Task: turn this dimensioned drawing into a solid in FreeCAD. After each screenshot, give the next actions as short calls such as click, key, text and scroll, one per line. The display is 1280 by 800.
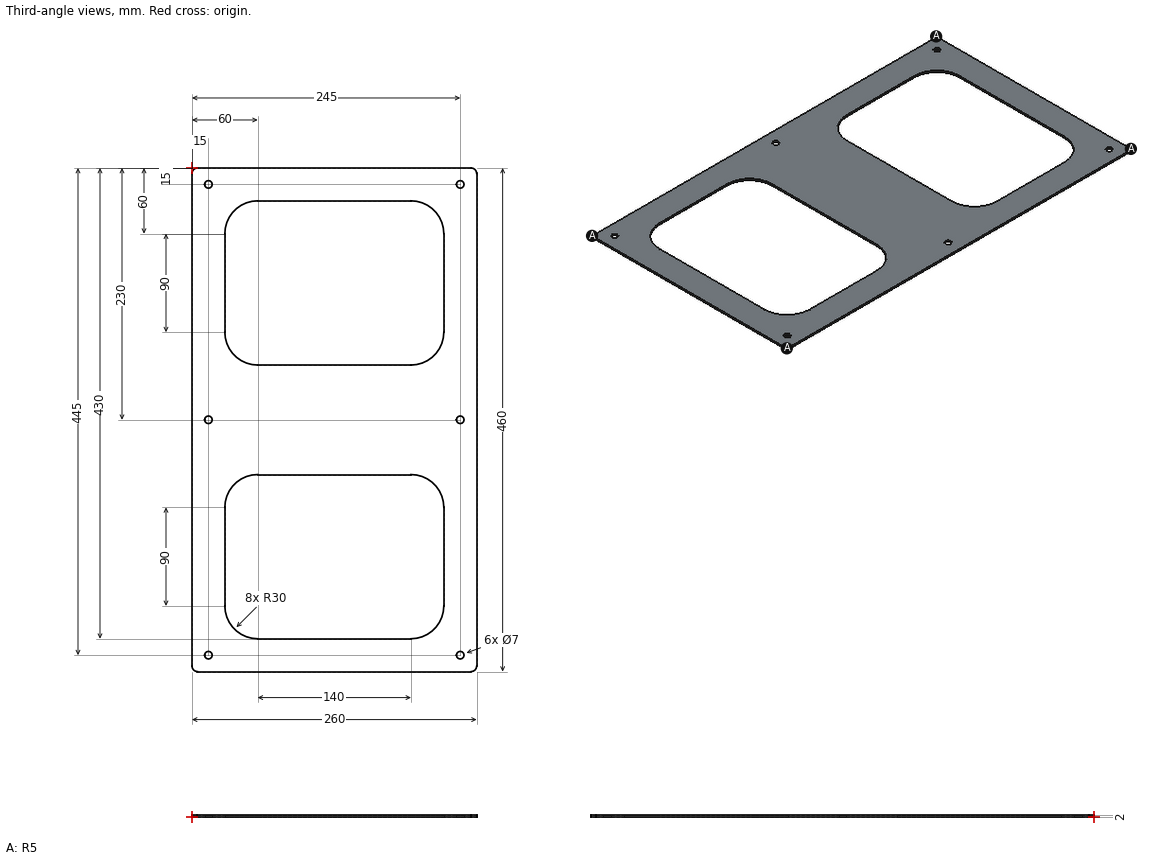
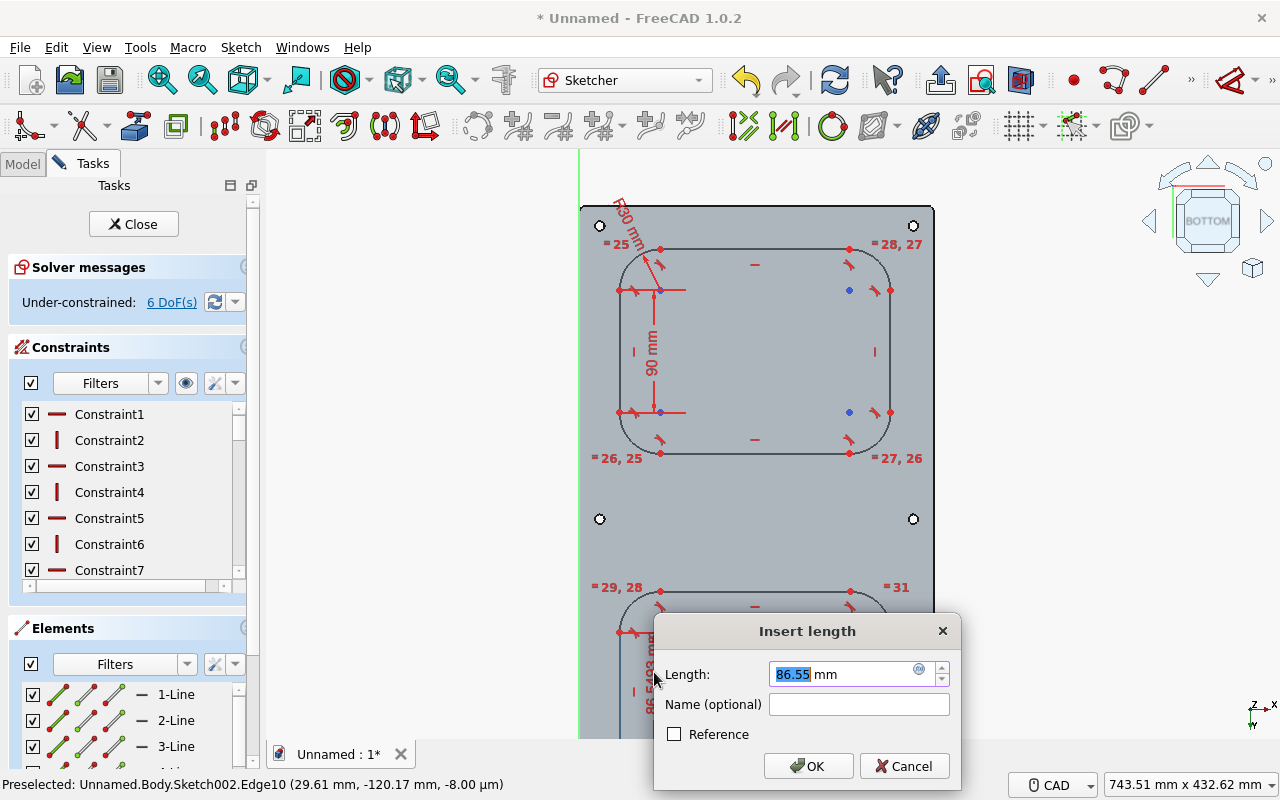
text(90)
key(Return)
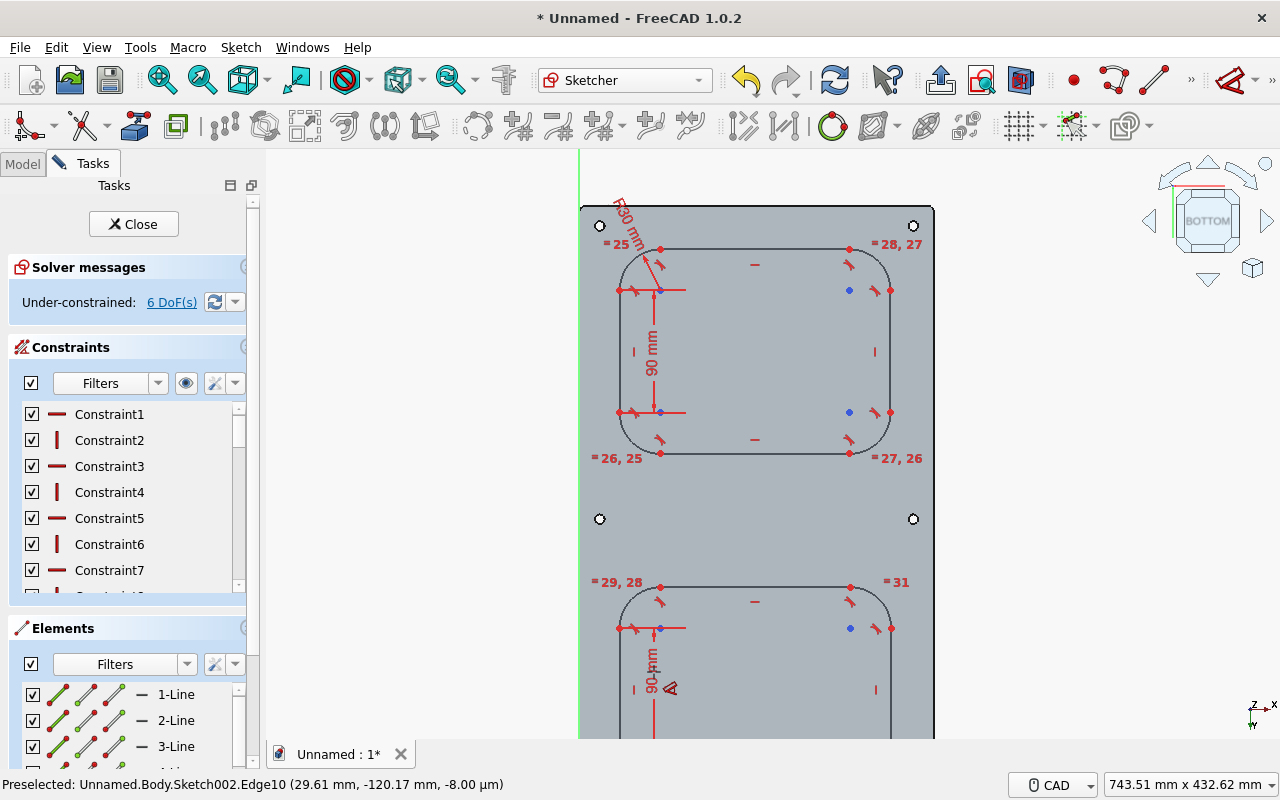
click(793, 249)
click(755, 215)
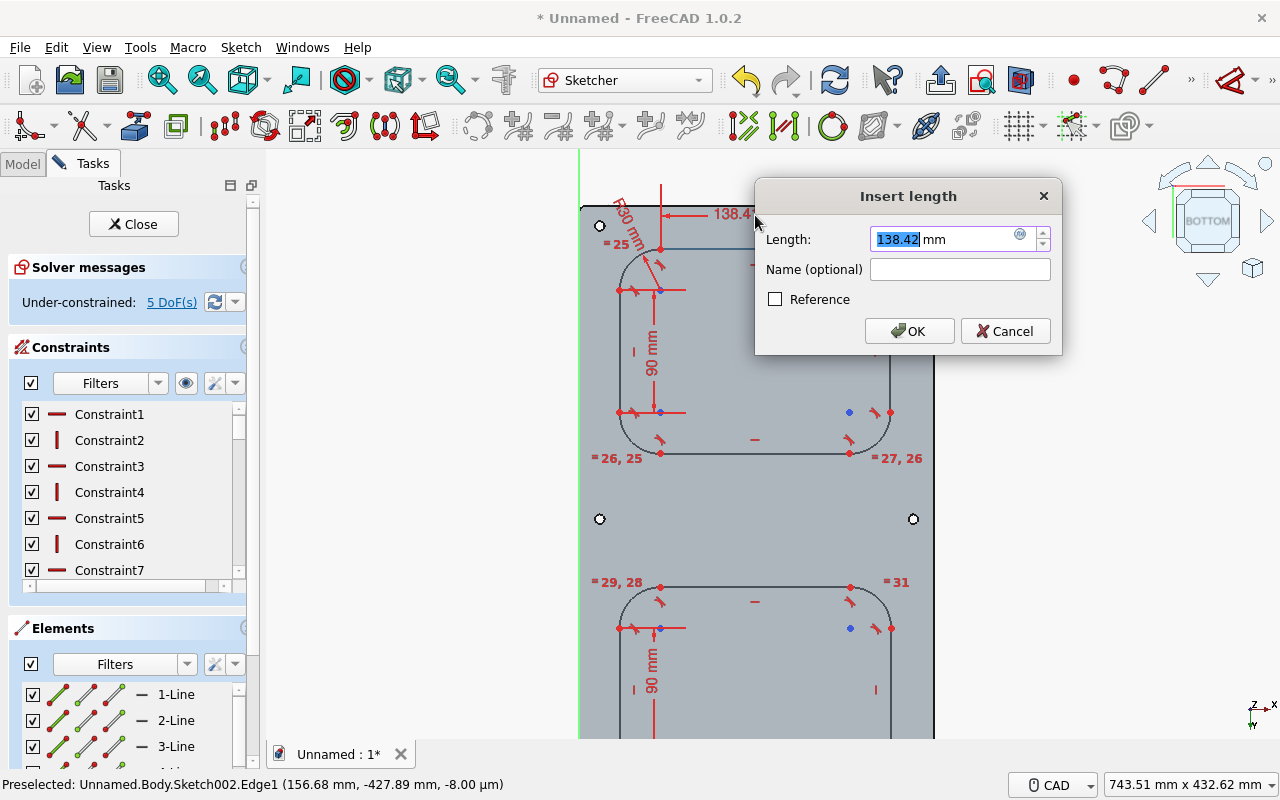
text(140)
key(Return)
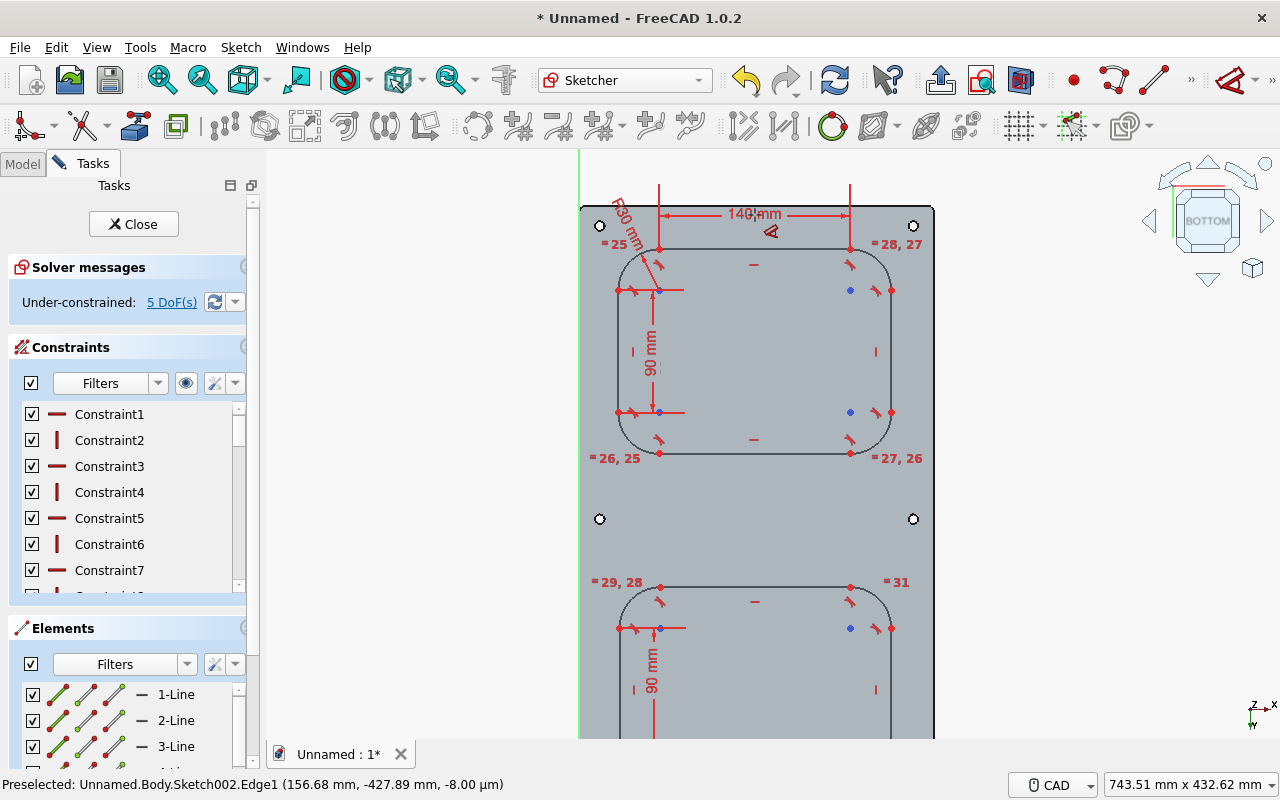
click(793, 587)
click(755, 621)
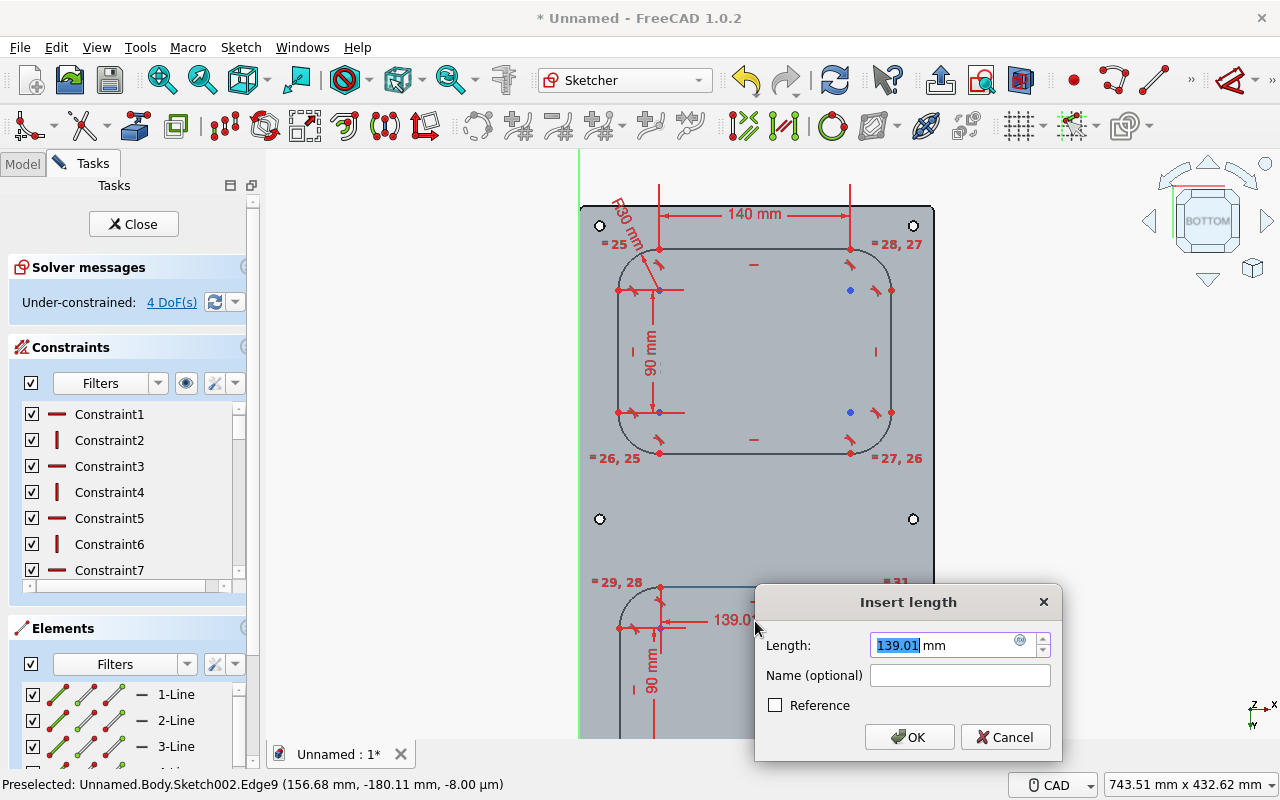
text(140)
key(Return)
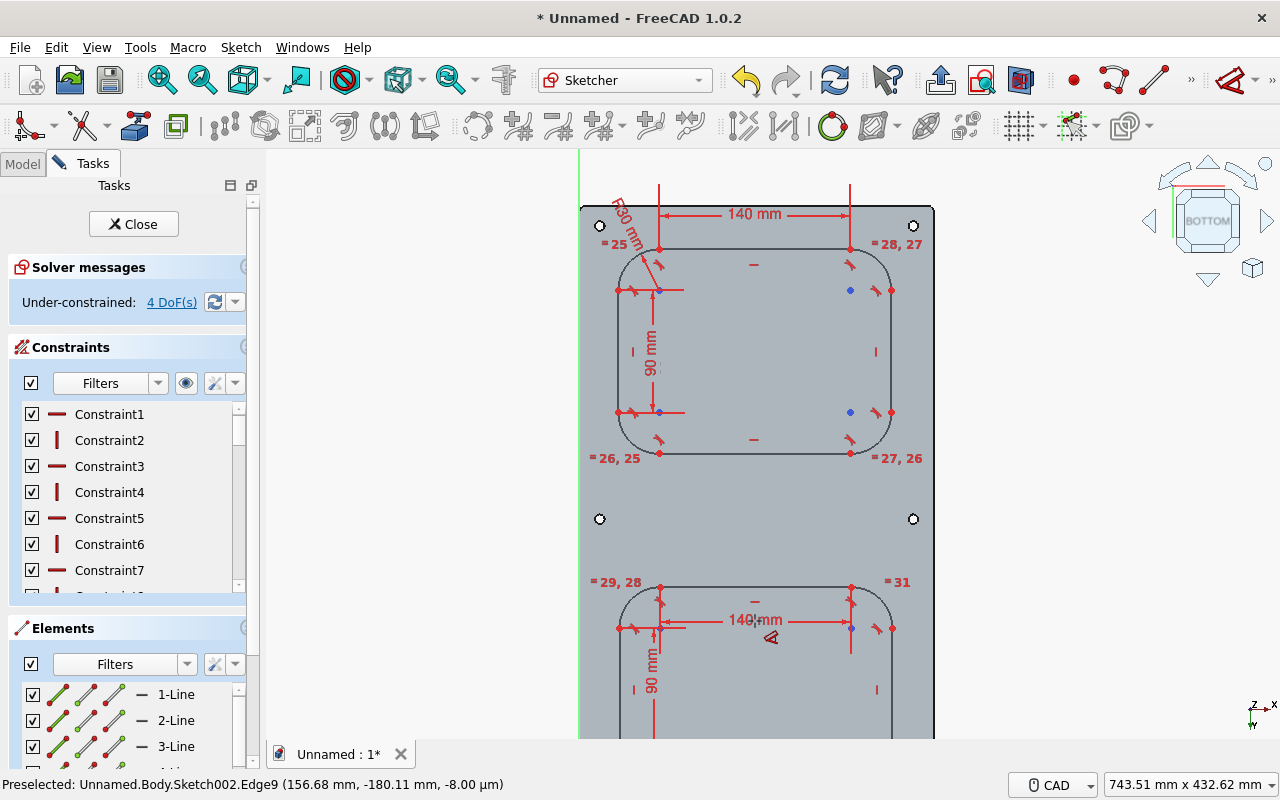
click(659, 249)
click(619, 191)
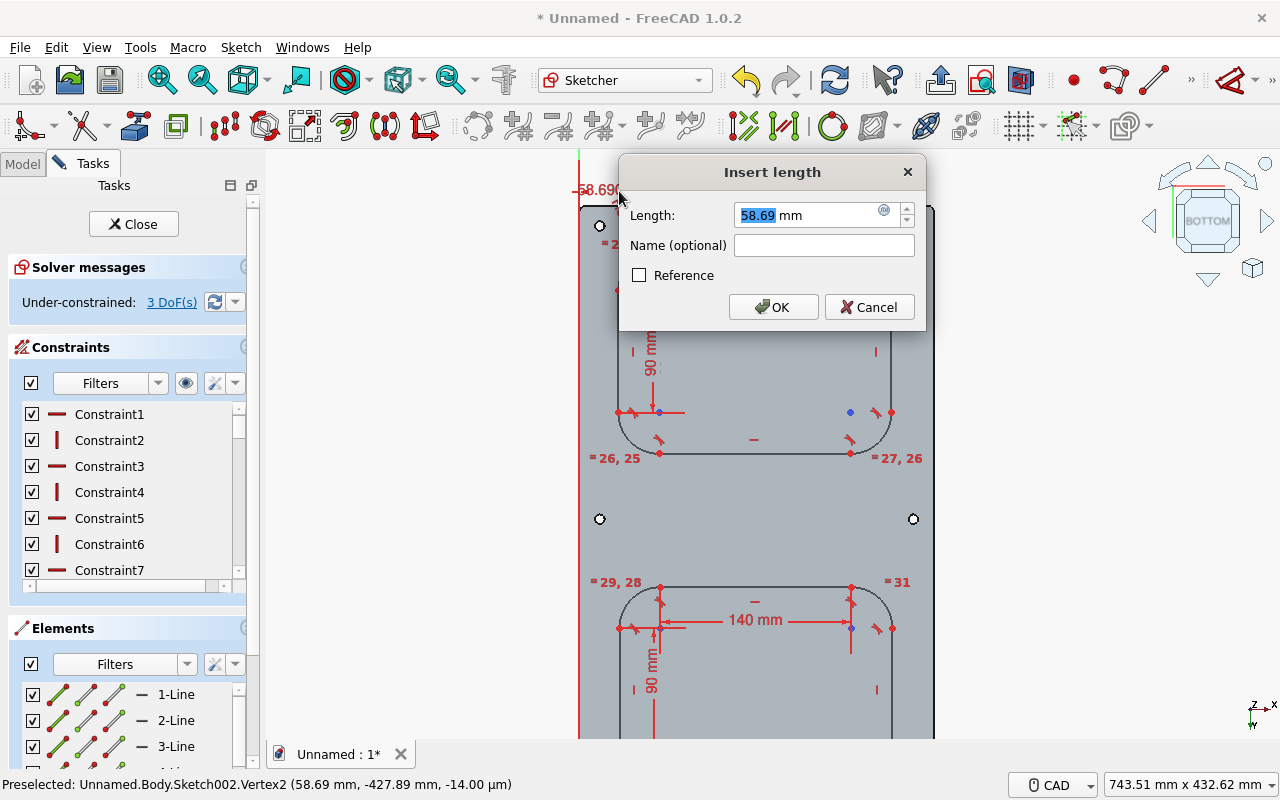
text(60)
key(Return)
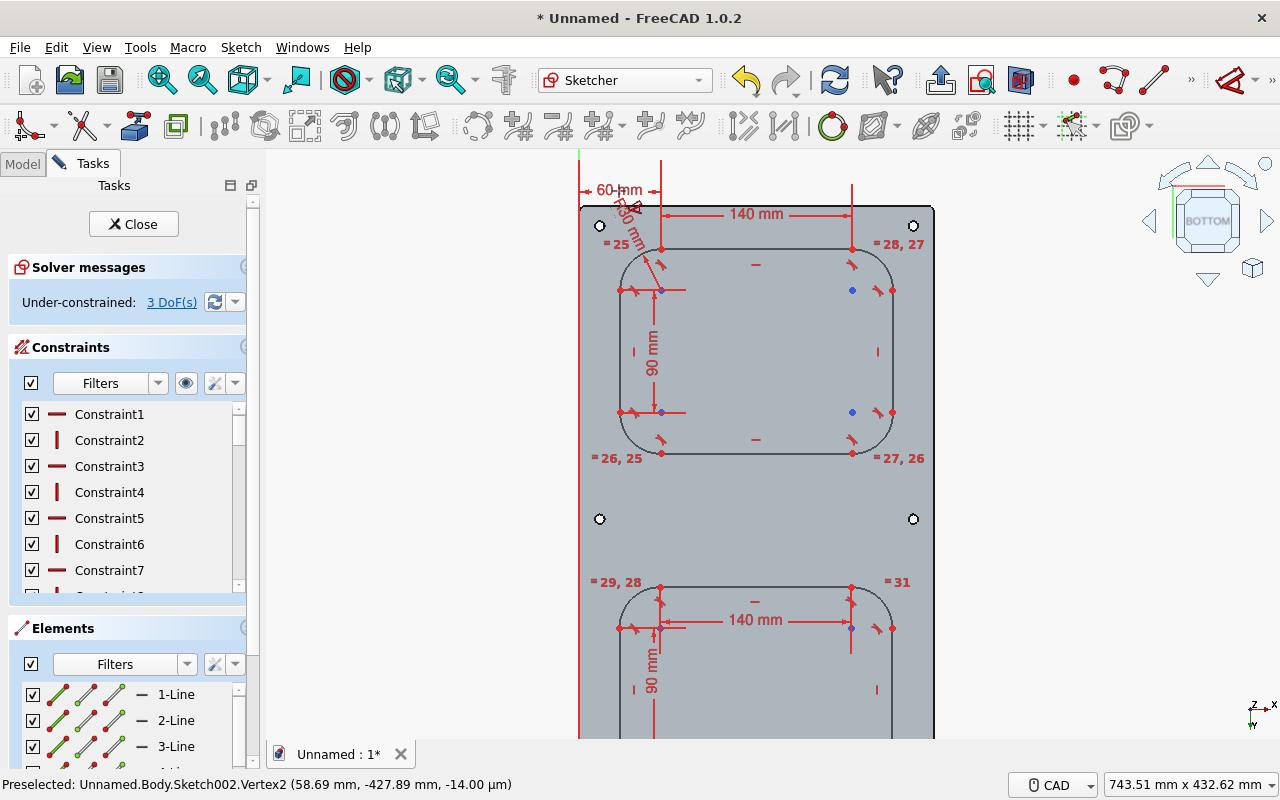
click(660, 587)
click(620, 553)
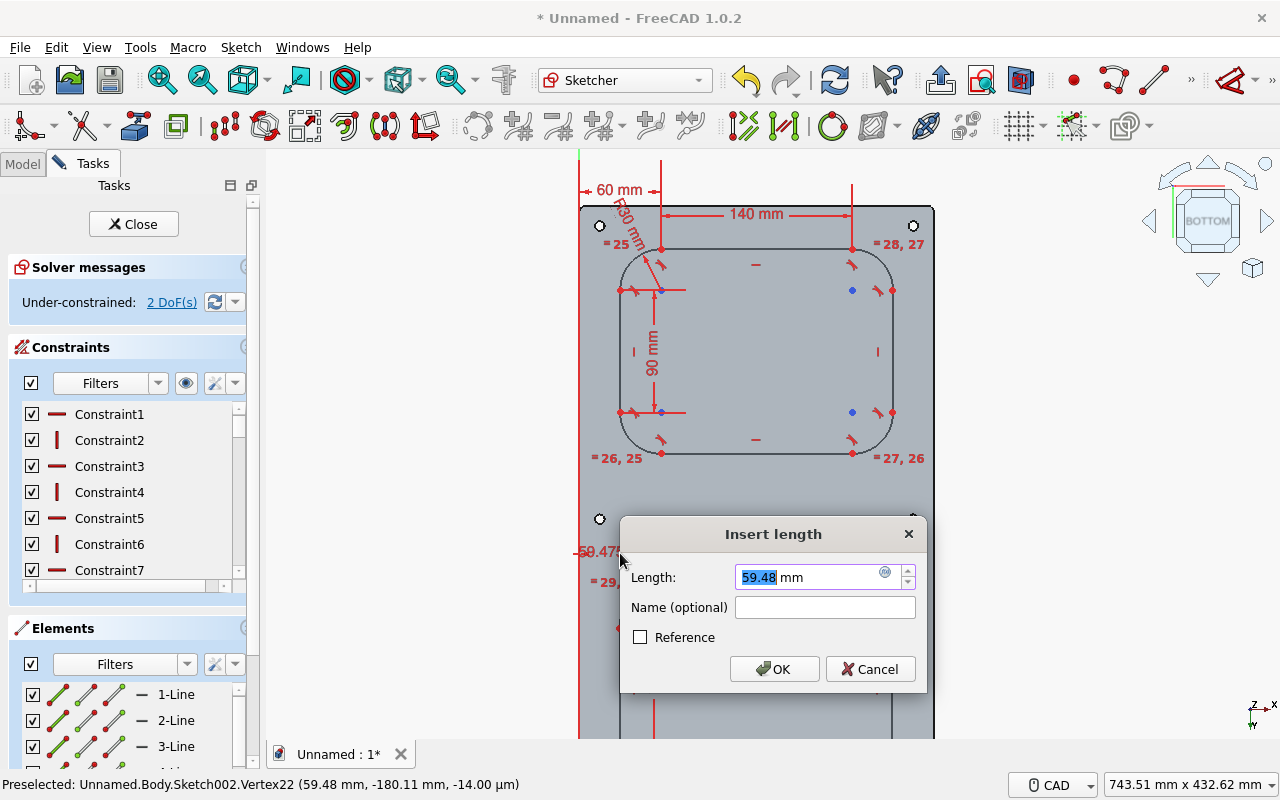
text(60)
key(Return)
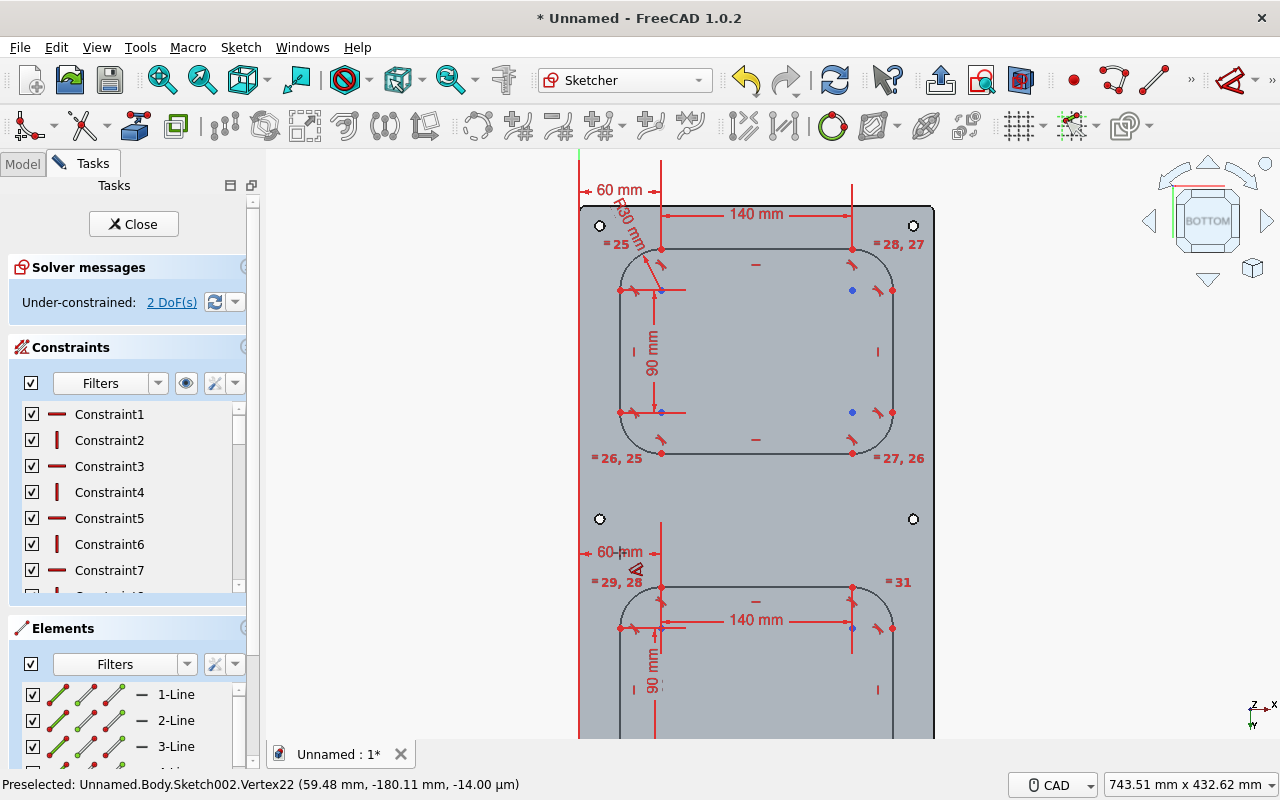
scroll(640, 249, down, 2)